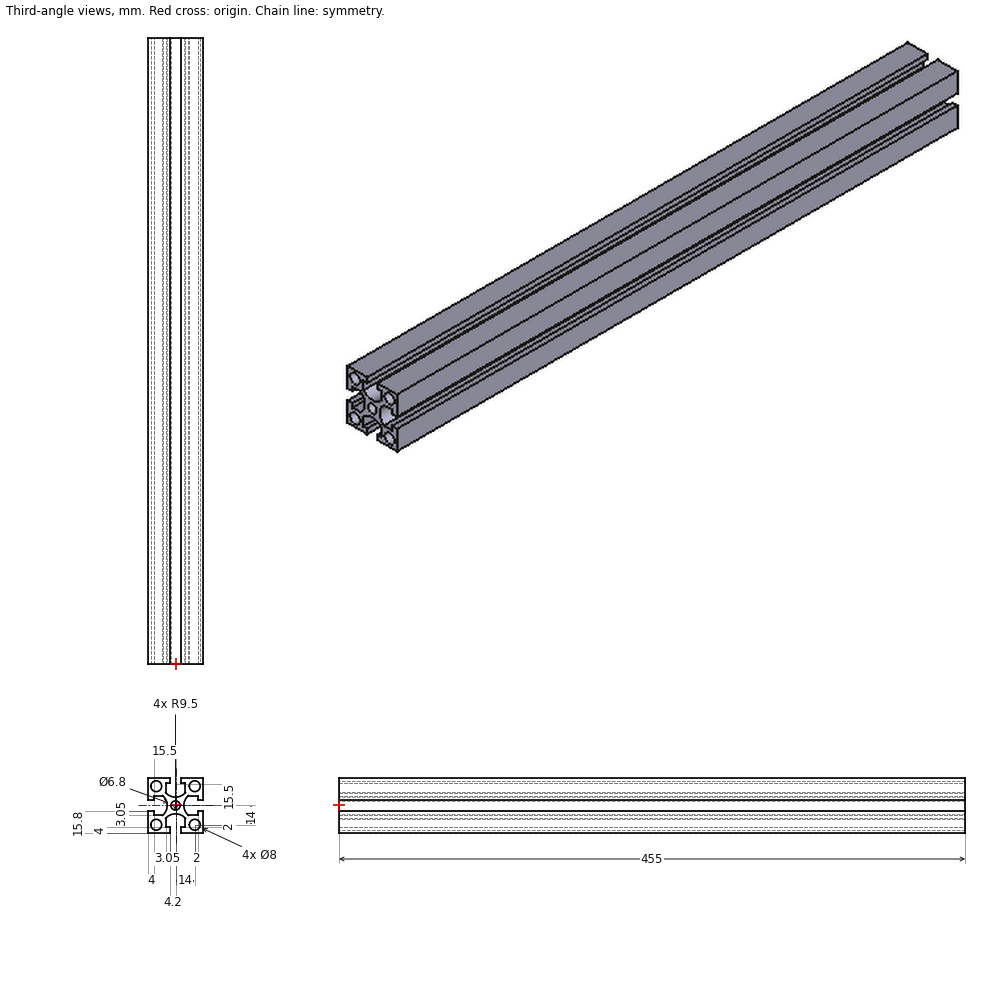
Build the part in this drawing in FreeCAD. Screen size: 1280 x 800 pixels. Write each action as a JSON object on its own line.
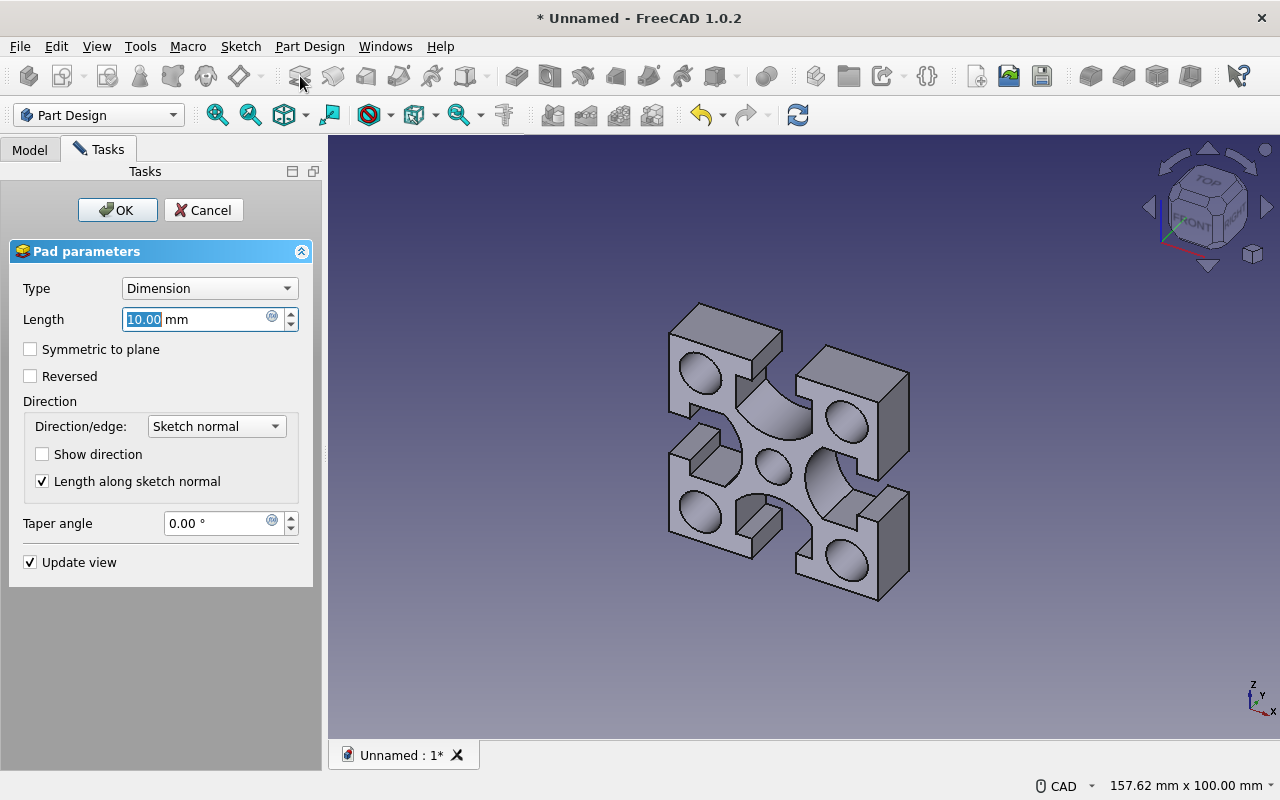
{"action": "type", "text": "455"}
{"action": "key", "text": "Tab"}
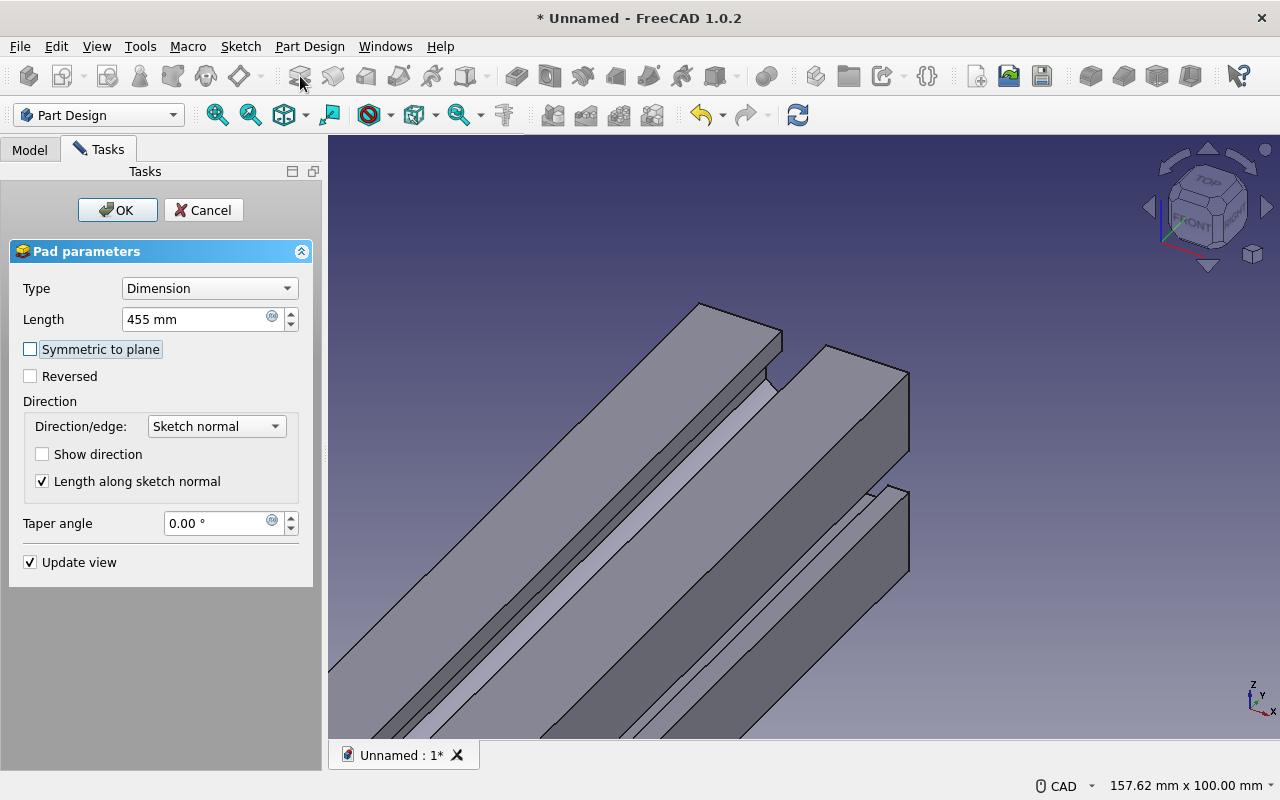
{"action": "left_click", "coordinate": [31, 376]}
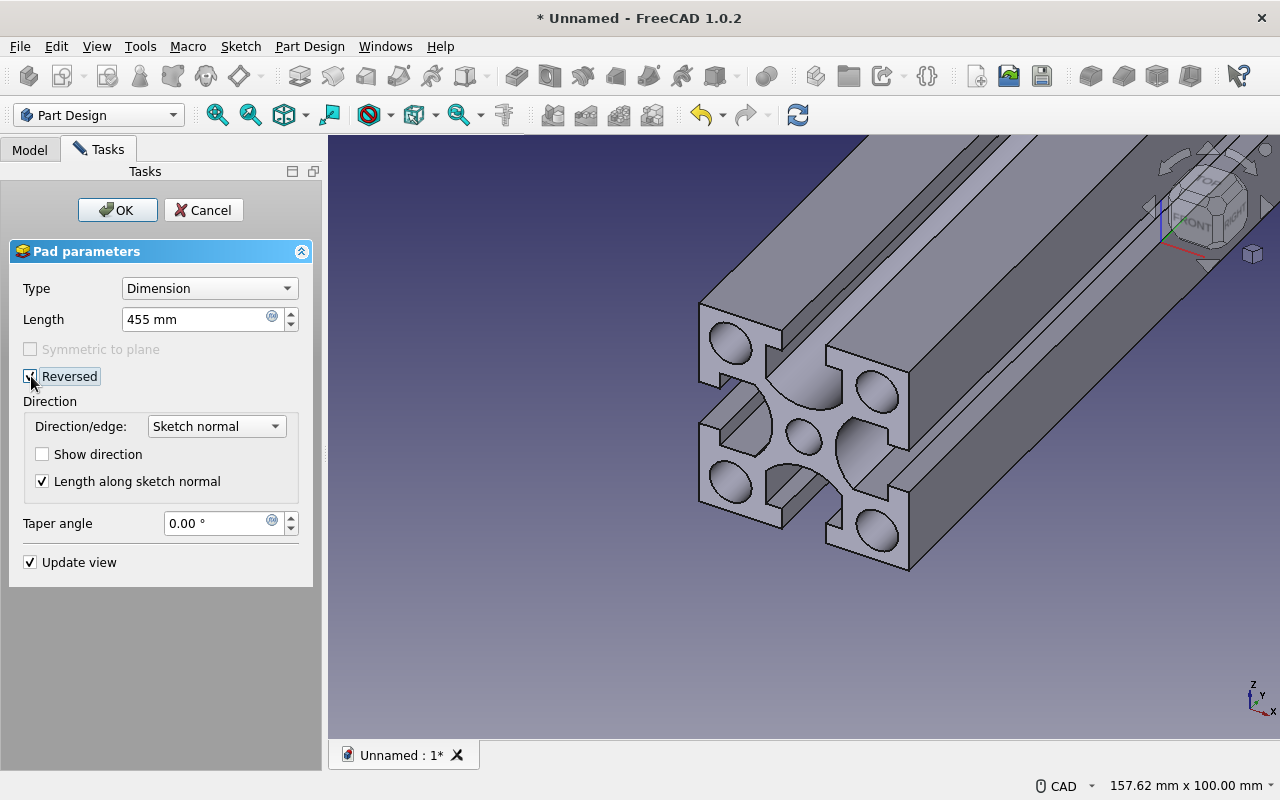
{"action": "left_click", "coordinate": [118, 210]}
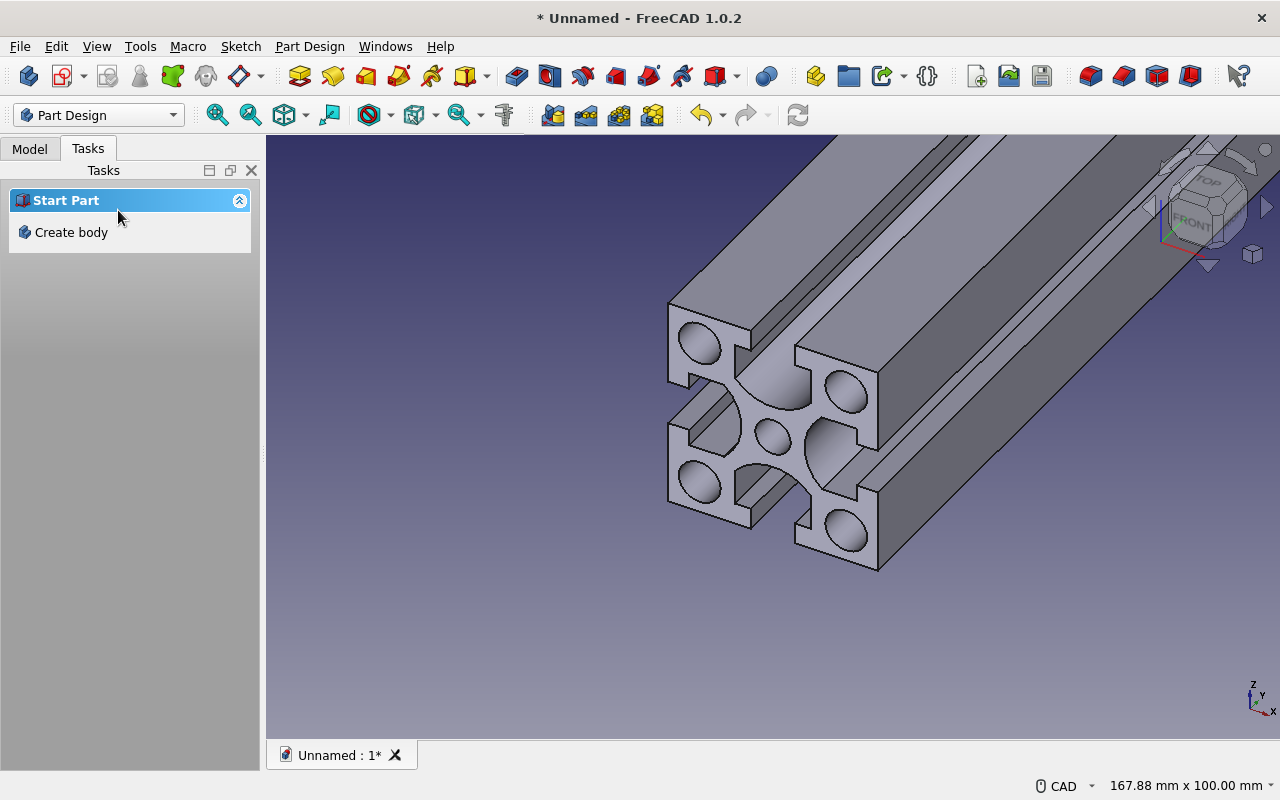
{"action": "key", "text": "0"}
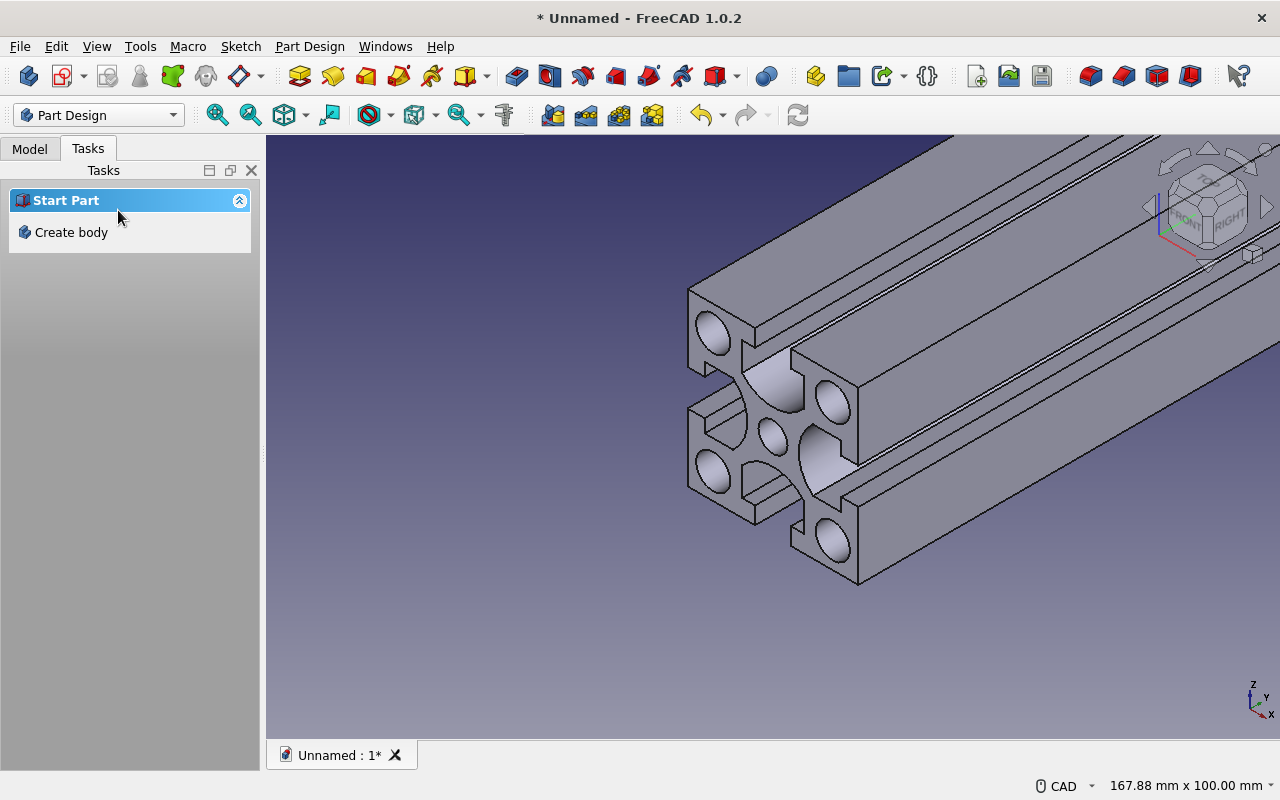
{"action": "left_click", "coordinate": [218, 116]}